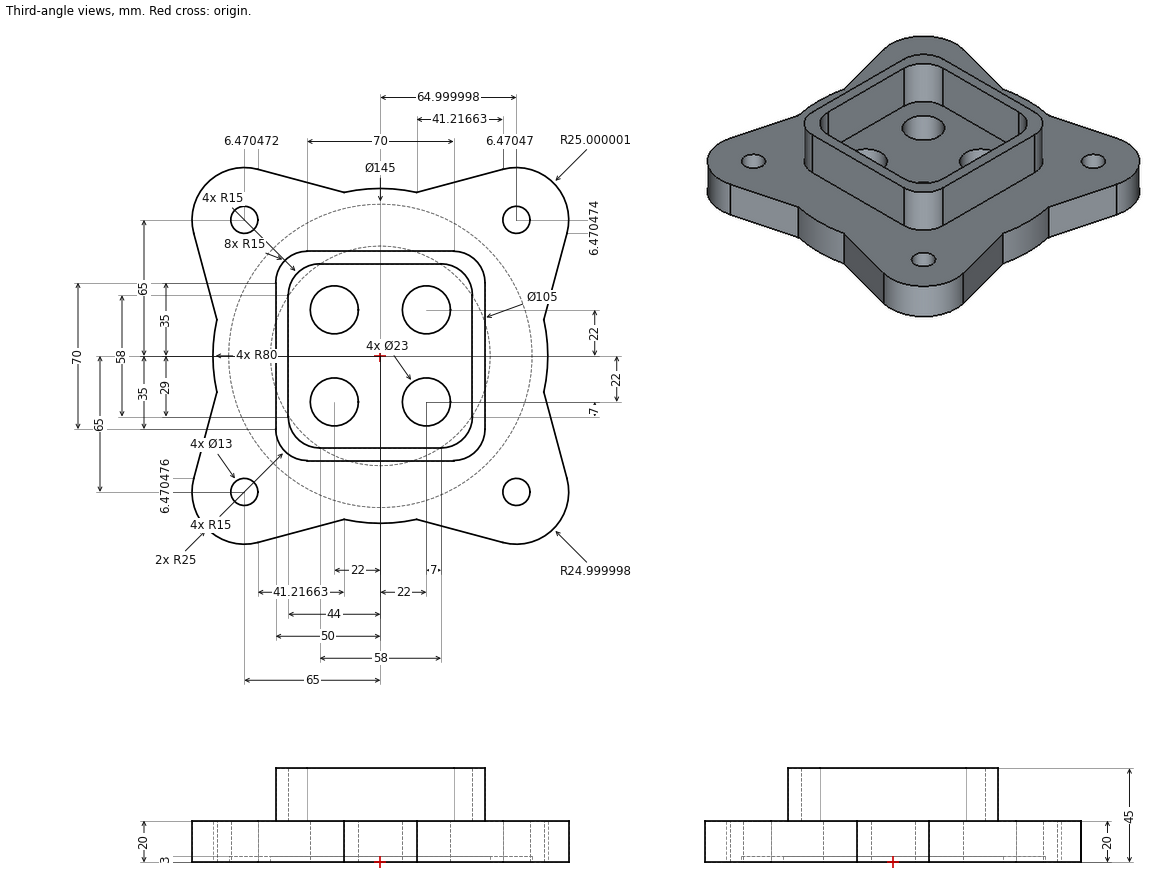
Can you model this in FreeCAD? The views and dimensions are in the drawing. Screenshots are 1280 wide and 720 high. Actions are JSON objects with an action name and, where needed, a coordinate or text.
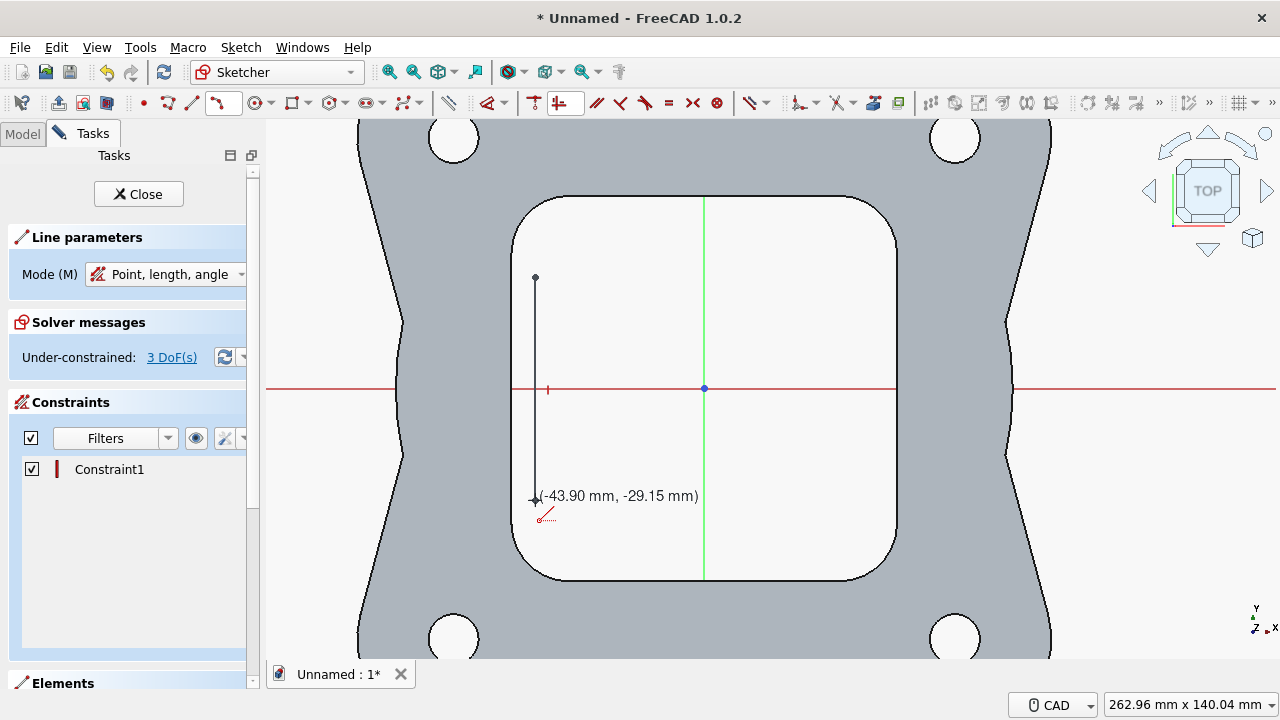
{"action": "left_click", "coordinate": [592, 558]}
{"action": "left_click", "coordinate": [816, 558]}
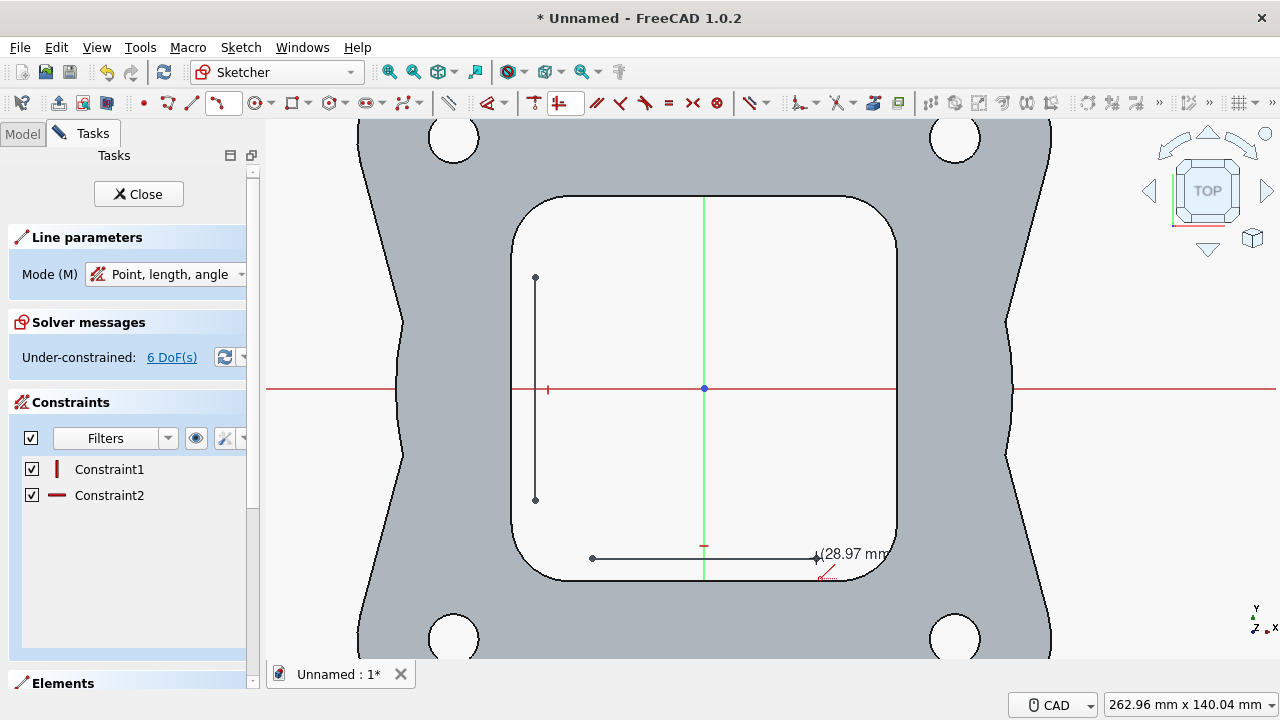
{"action": "left_click", "coordinate": [874, 500]}
{"action": "left_click", "coordinate": [874, 277]}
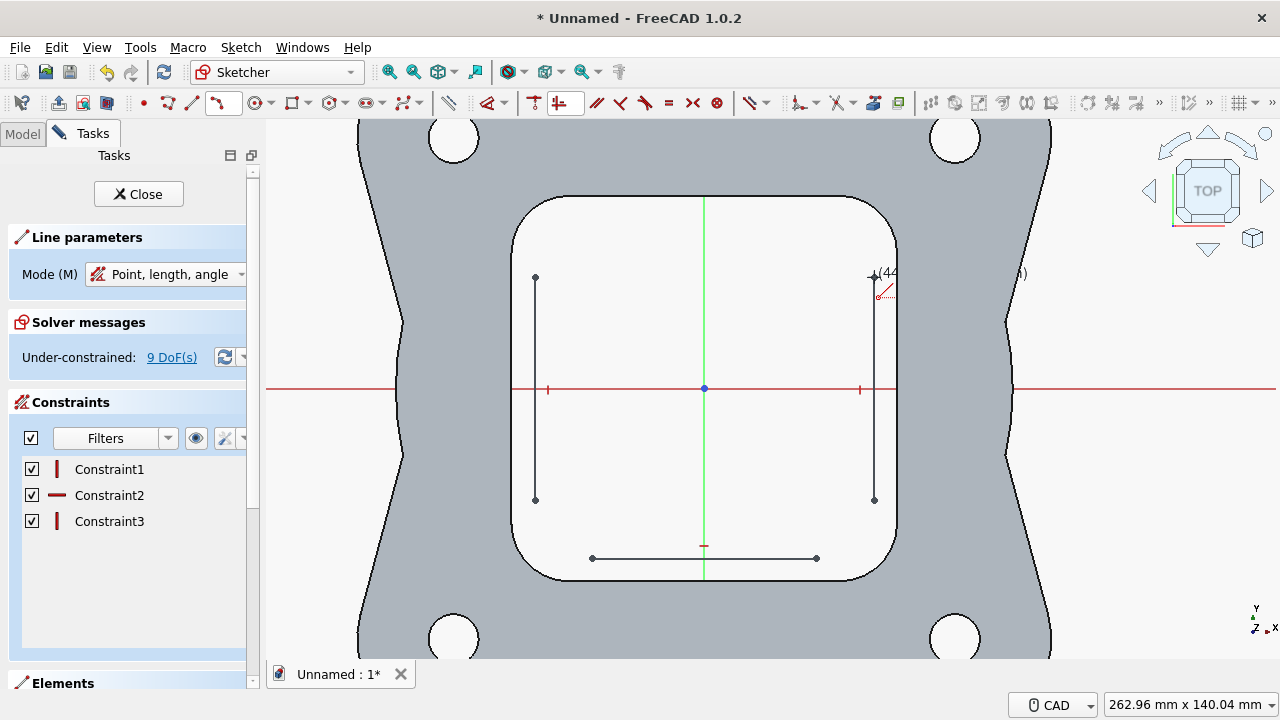
{"action": "left_click", "coordinate": [816, 219]}
{"action": "left_click", "coordinate": [592, 219]}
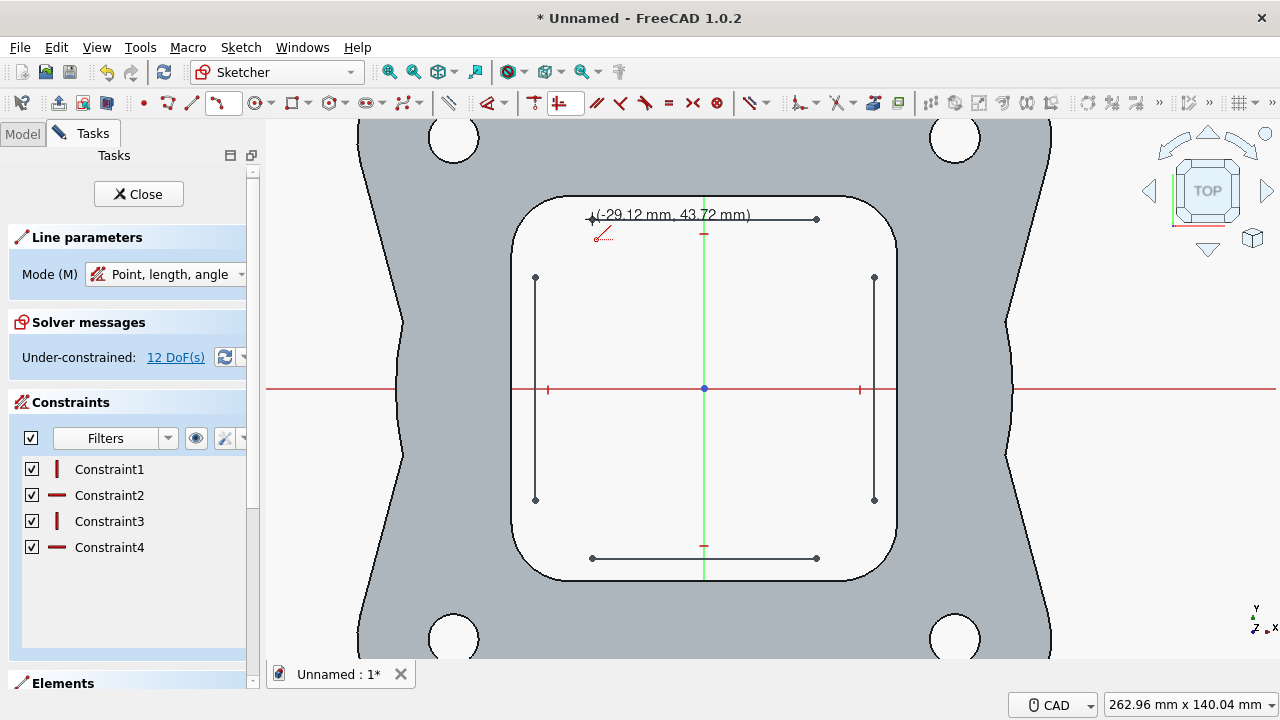
{"action": "left_click", "coordinate": [218, 104]}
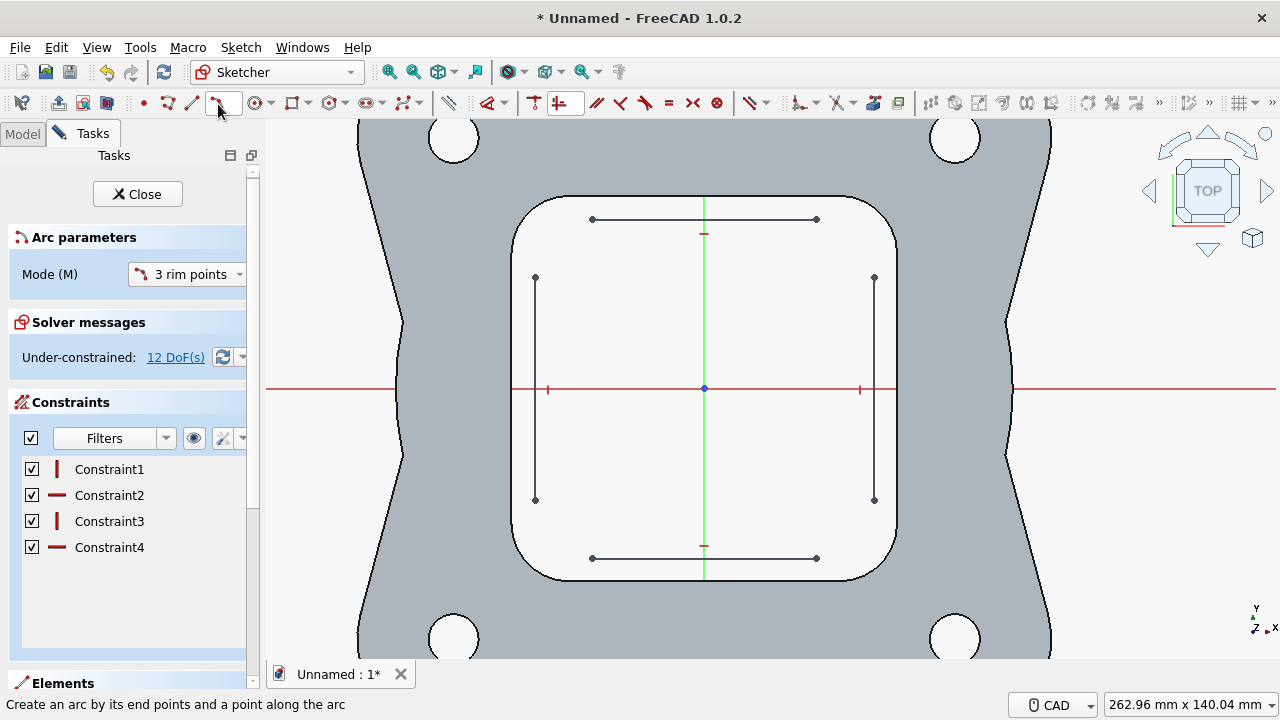
{"action": "left_click", "coordinate": [535, 501]}
{"action": "left_click", "coordinate": [592, 559]}
{"action": "left_click", "coordinate": [552, 541]}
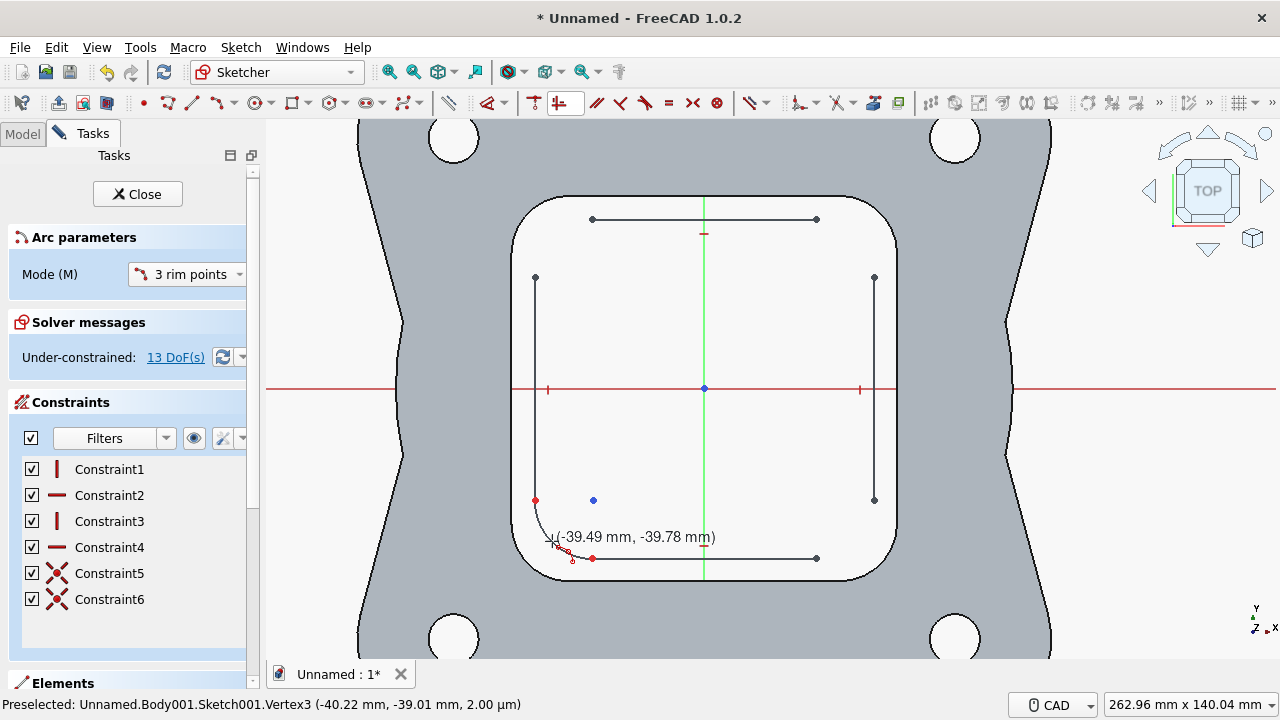
{"action": "left_click", "coordinate": [816, 559]}
{"action": "left_click", "coordinate": [874, 501]}
{"action": "left_click", "coordinate": [857, 541]}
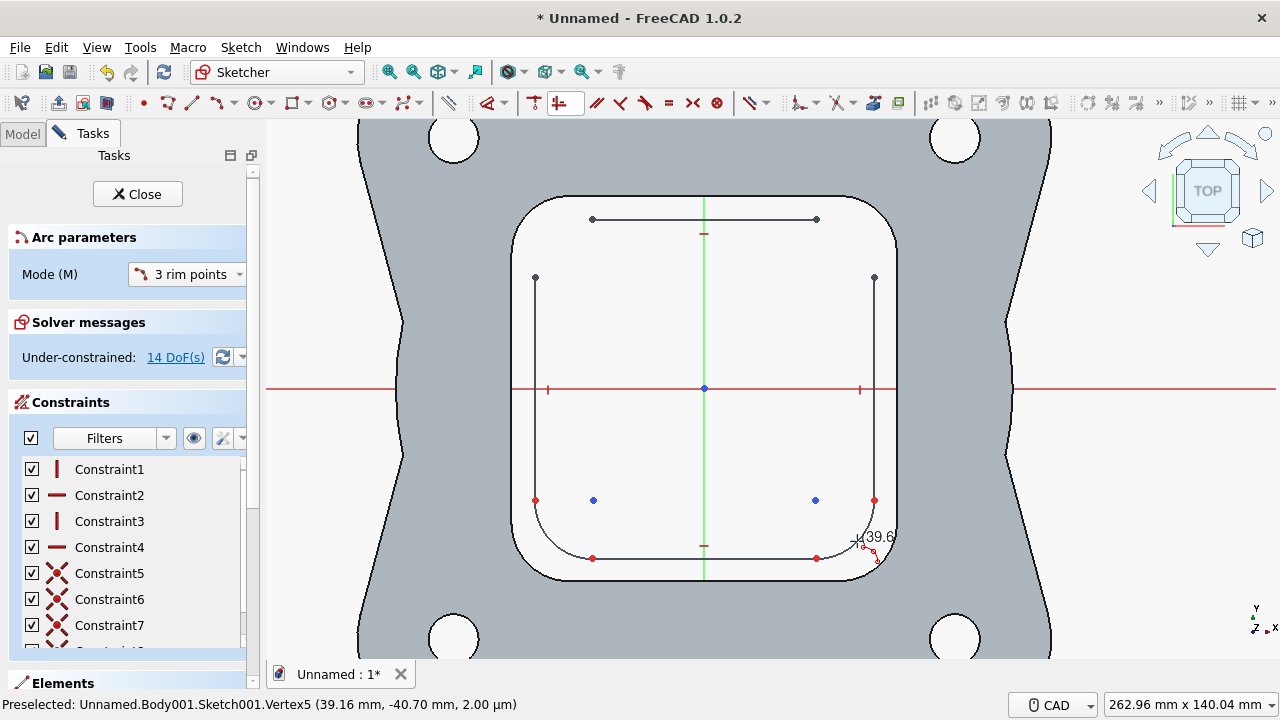
{"action": "left_click", "coordinate": [874, 278]}
{"action": "left_click", "coordinate": [816, 220]}
{"action": "left_click", "coordinate": [857, 236]}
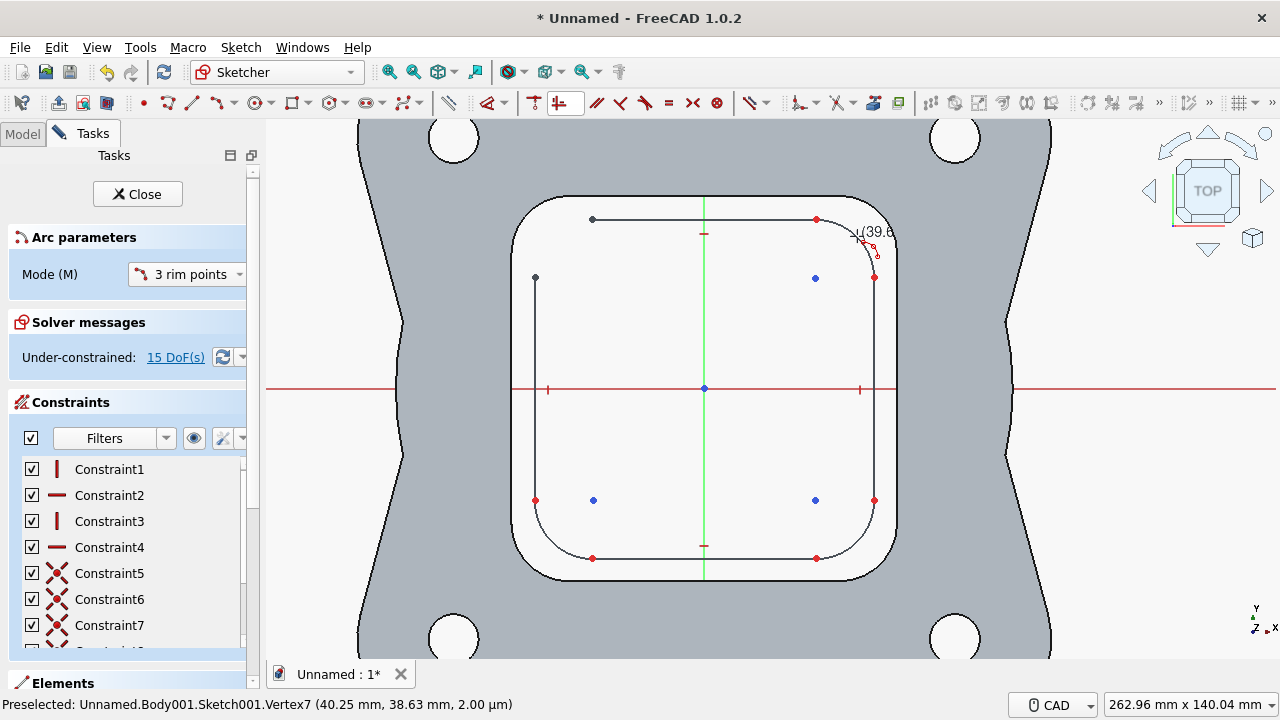
{"action": "left_click", "coordinate": [592, 220]}
{"action": "left_click", "coordinate": [535, 278]}
{"action": "left_click", "coordinate": [552, 236]}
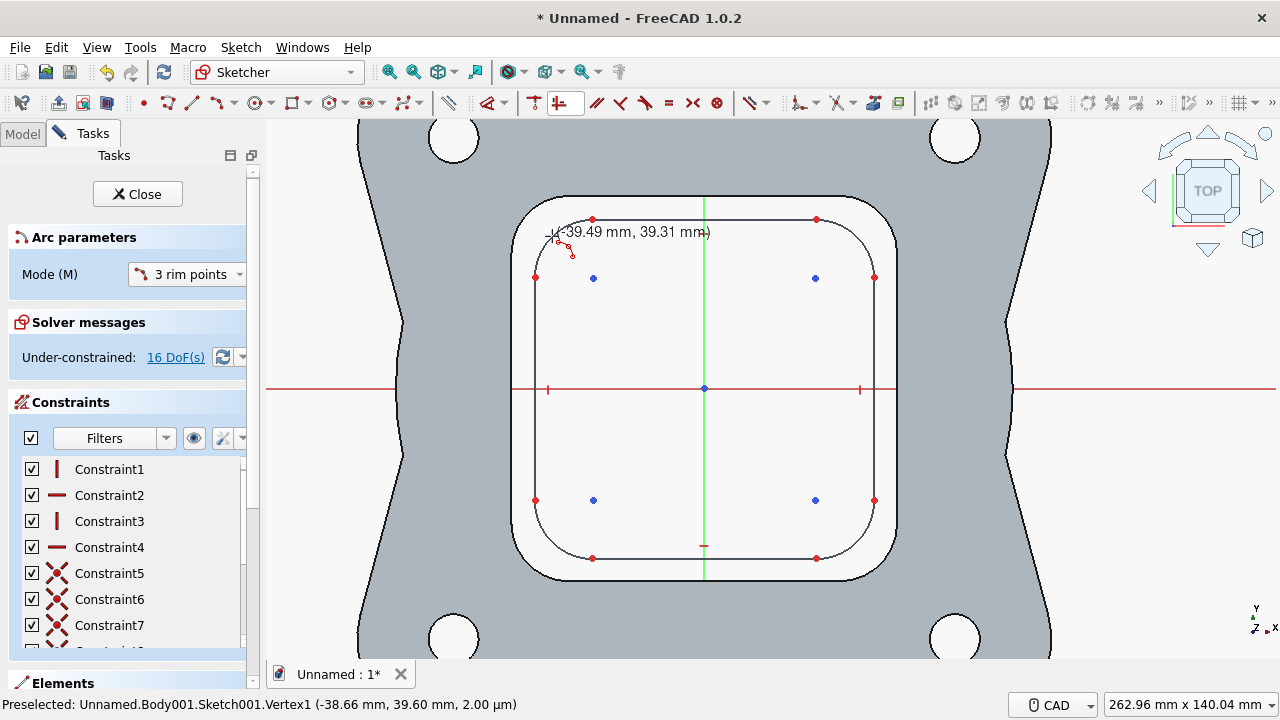
{"action": "left_click", "coordinate": [256, 104]}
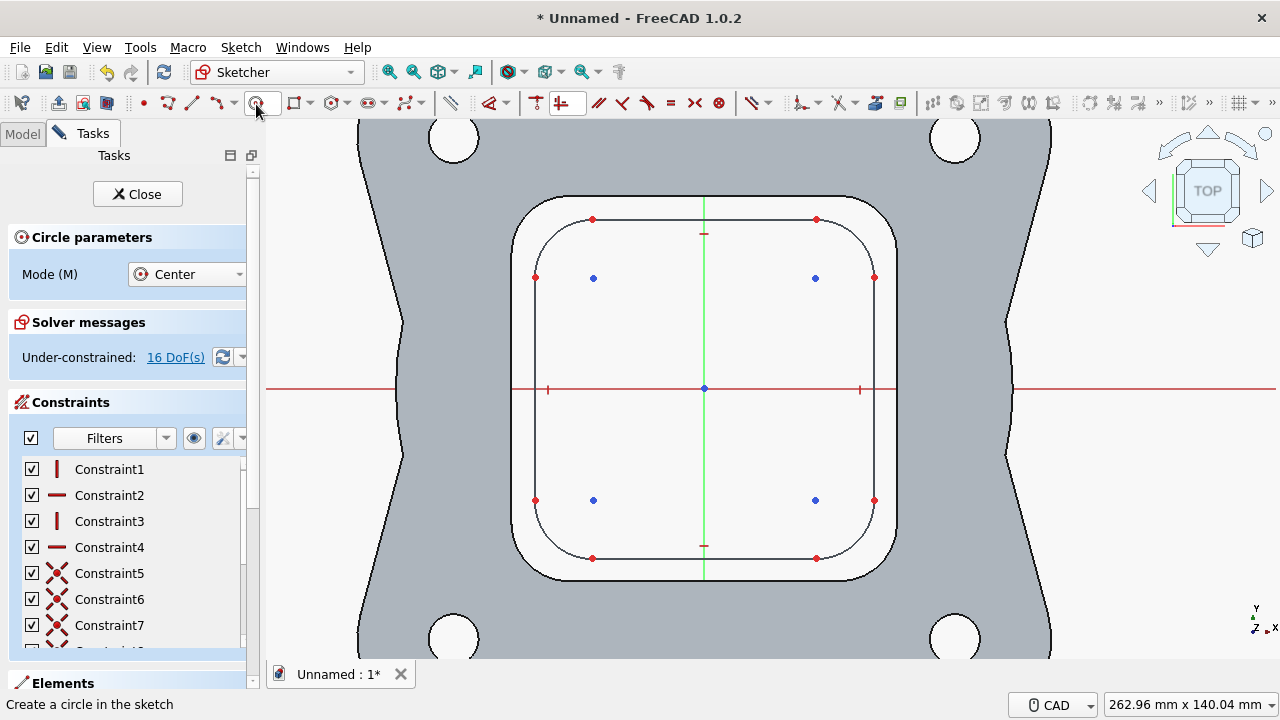
{"action": "left_click", "coordinate": [789, 473]}
{"action": "mouse_move", "coordinate": [820, 442]}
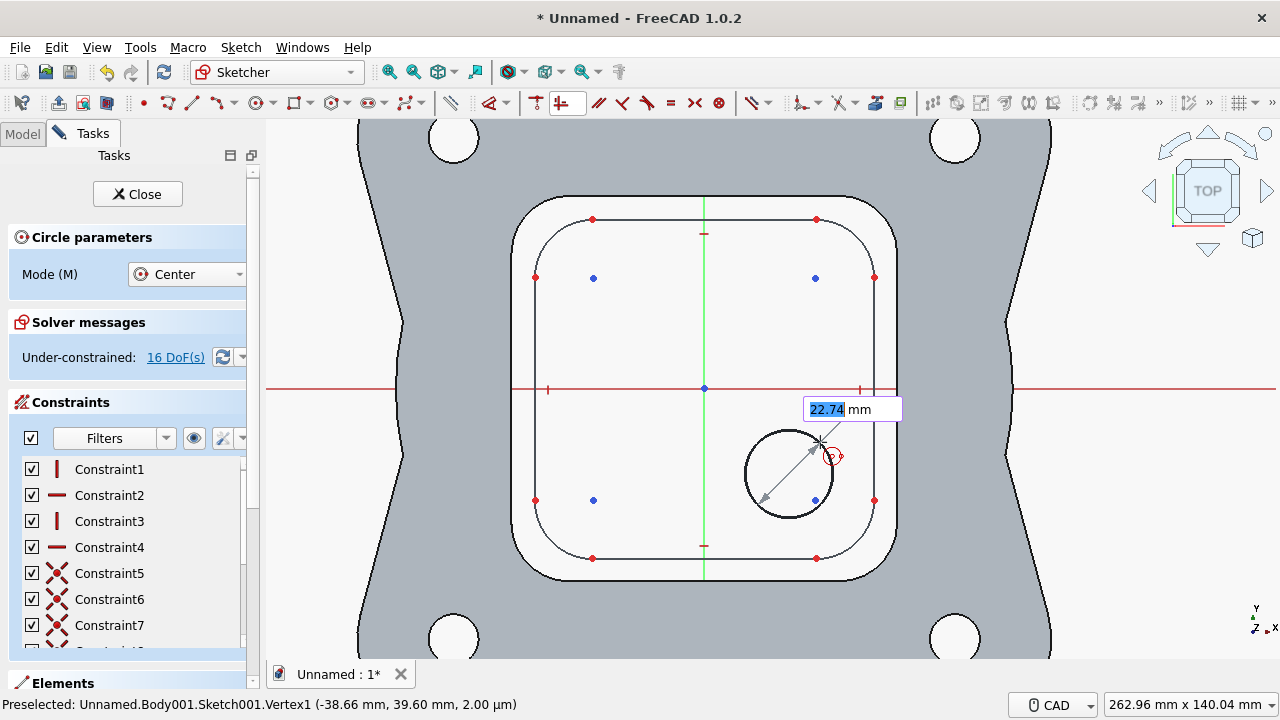
{"action": "type", "text": "23"}
{"action": "key", "text": "Return"}